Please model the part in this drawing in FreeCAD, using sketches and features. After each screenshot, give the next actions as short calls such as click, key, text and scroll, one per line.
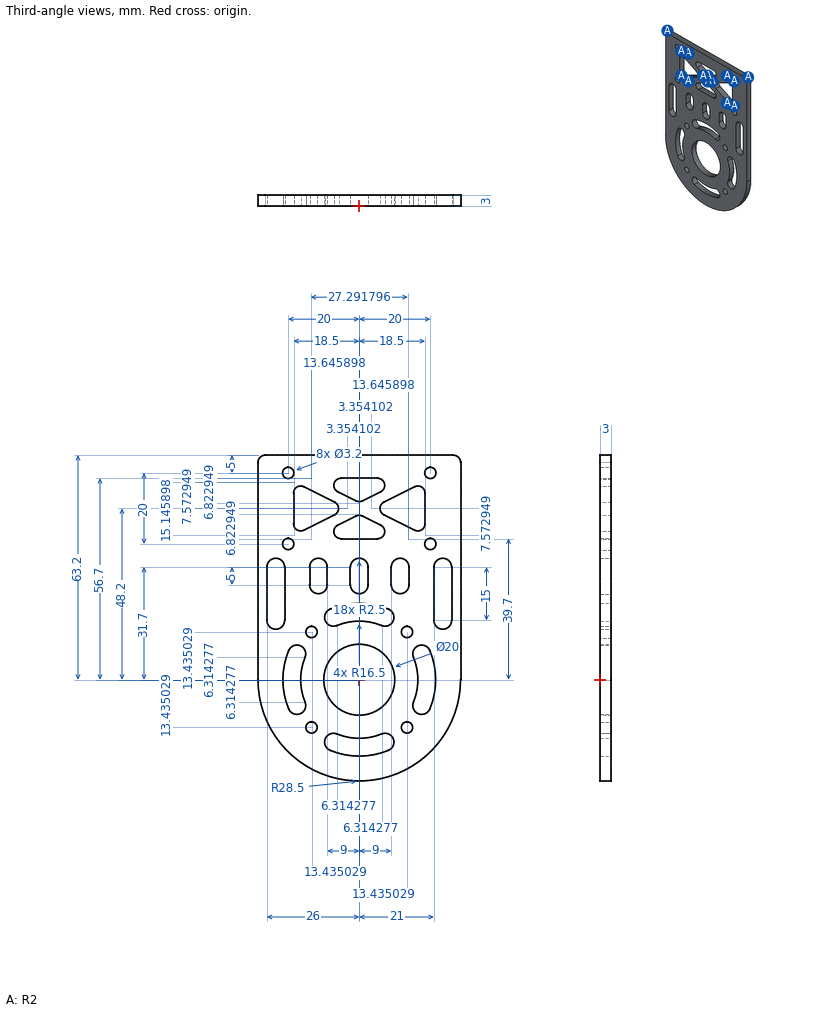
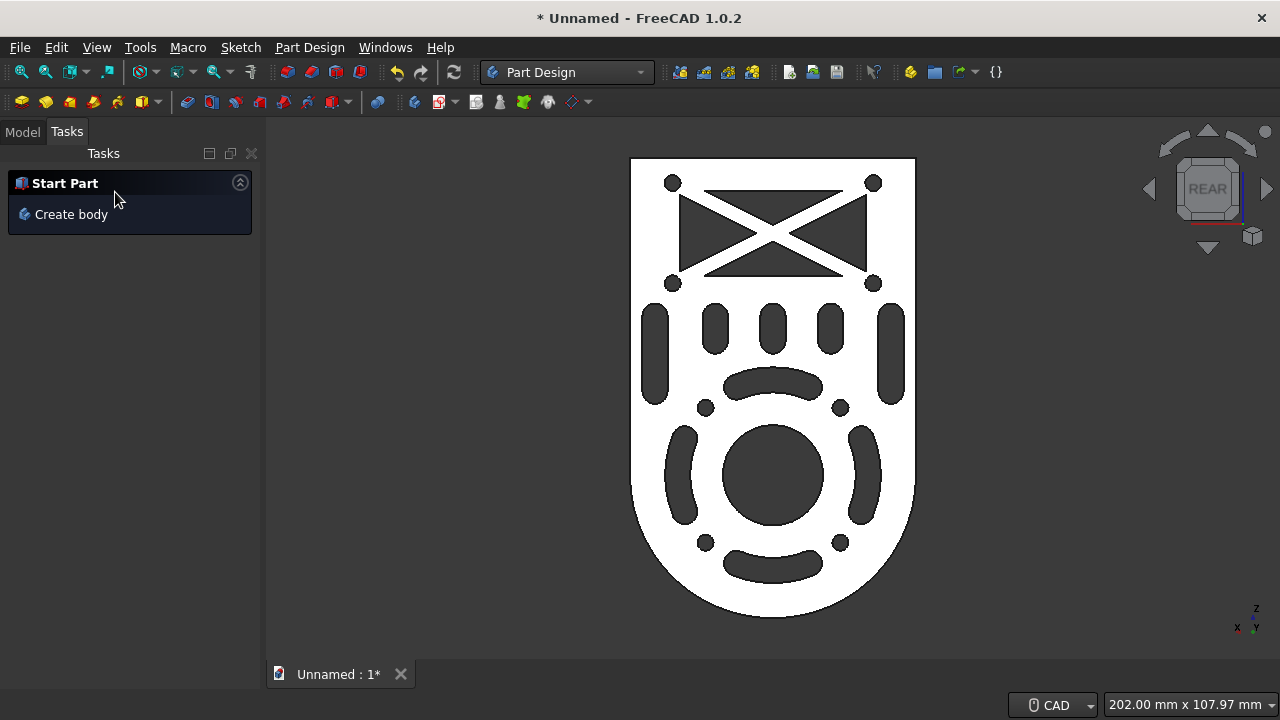
scroll(756, 232, up, 5)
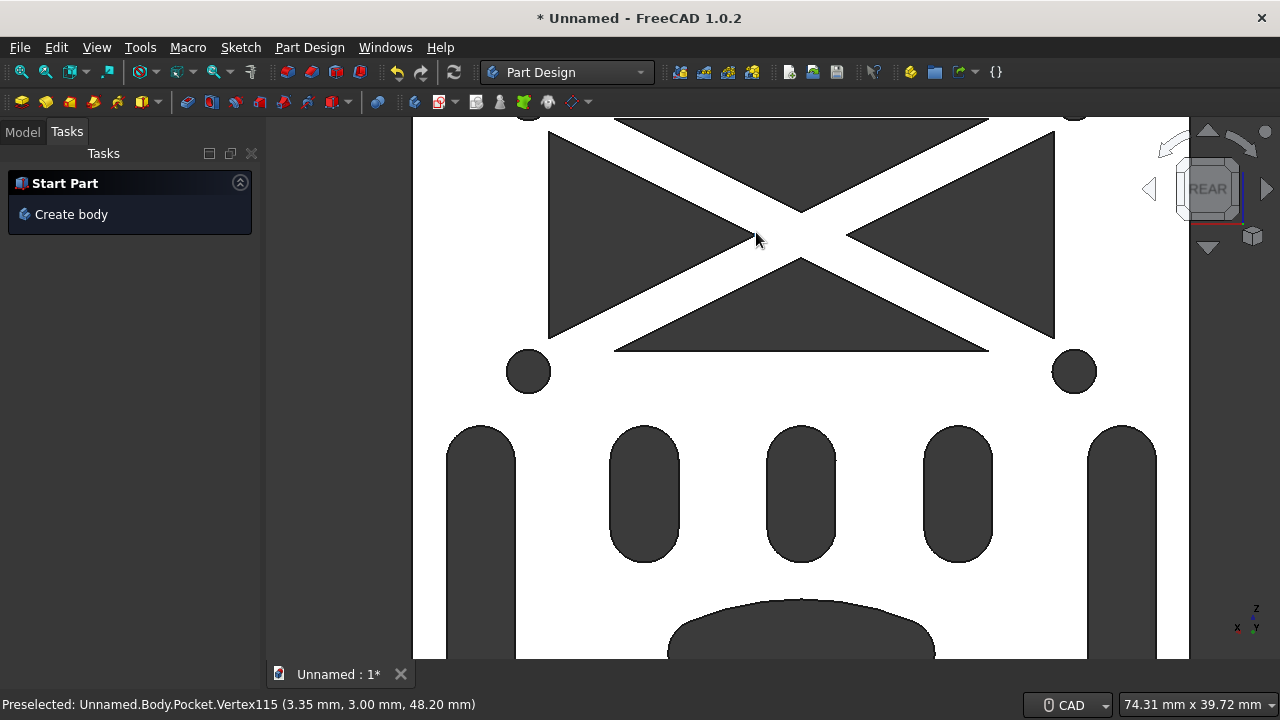
key(v)
key(f)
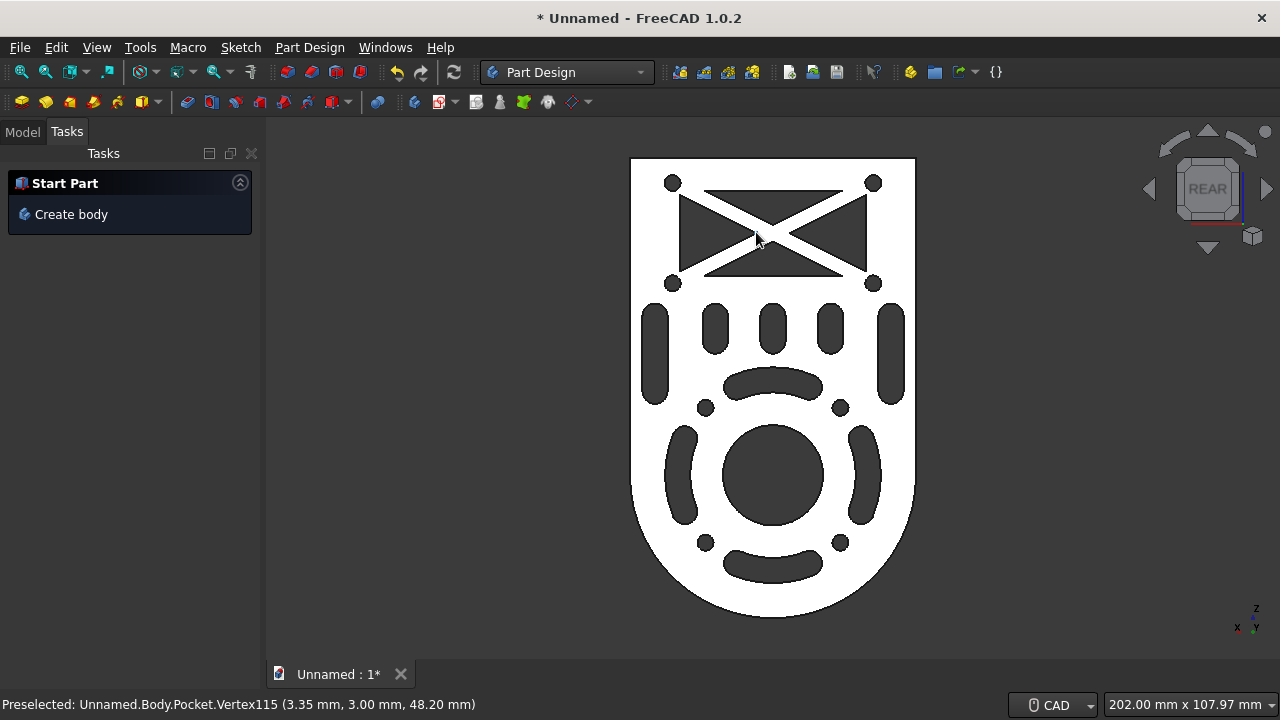
key(0)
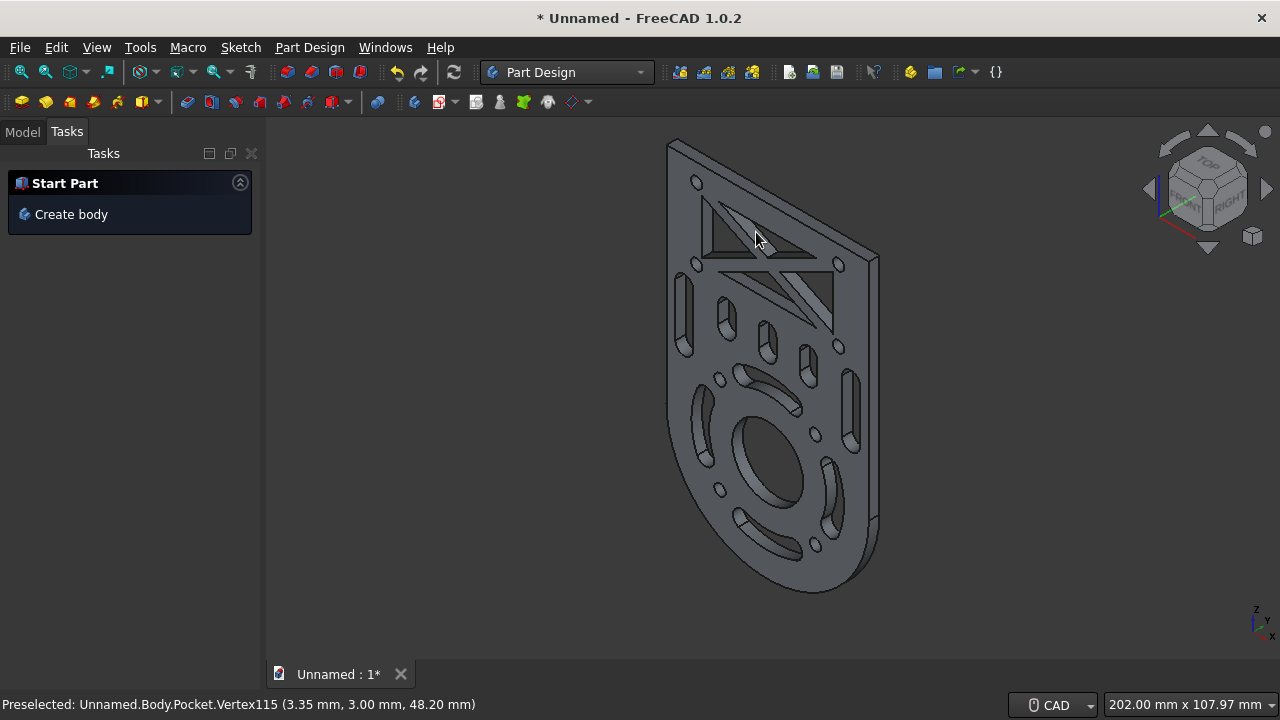
click(875, 257)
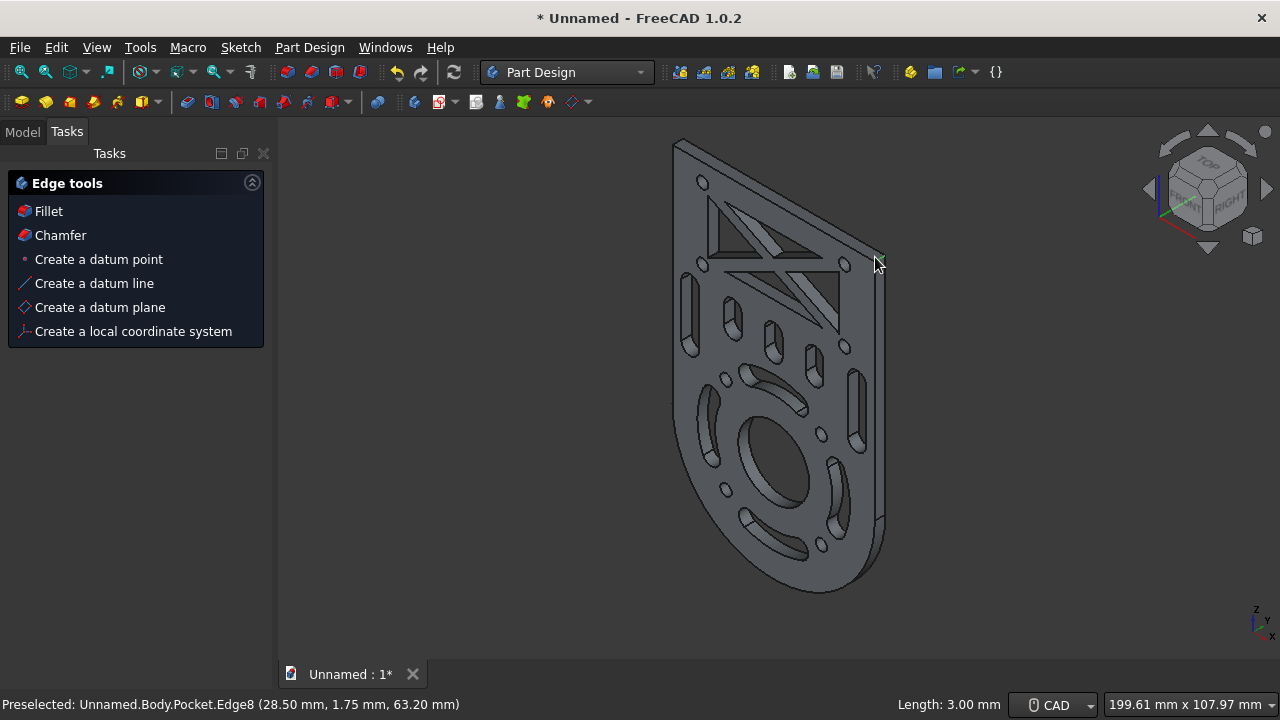
scroll(791, 268, up, 5)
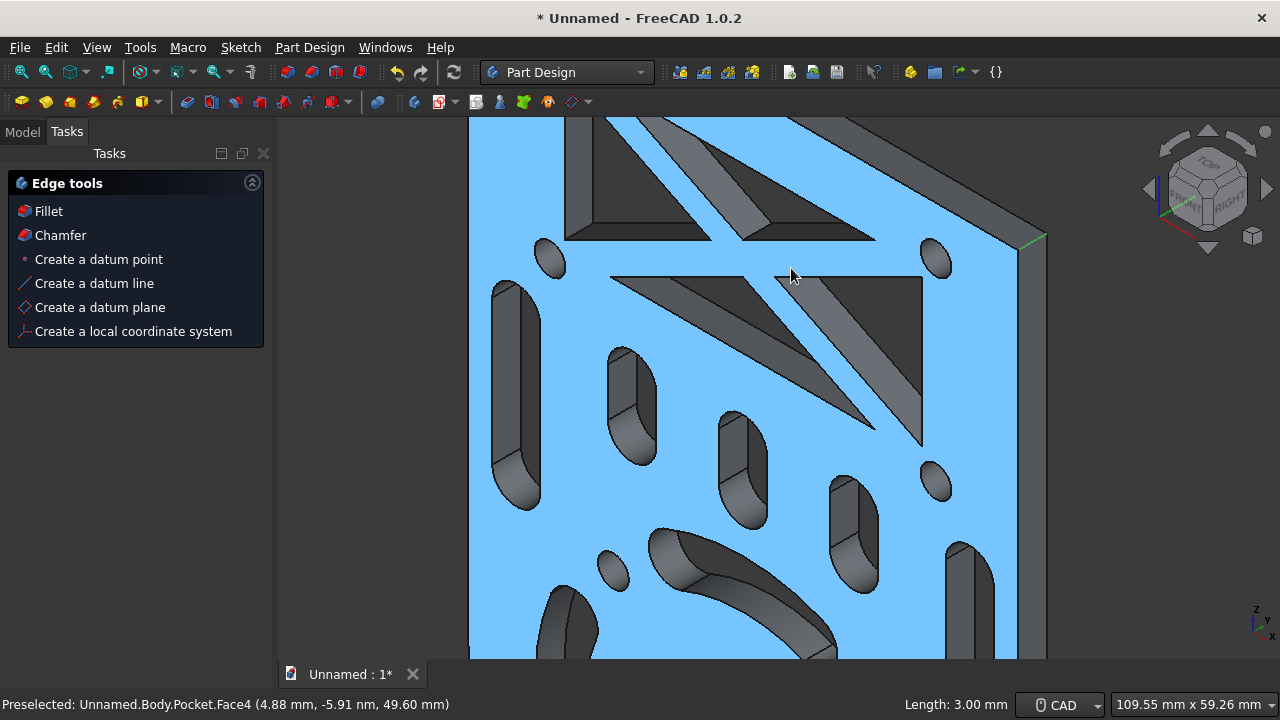
click(22, 72)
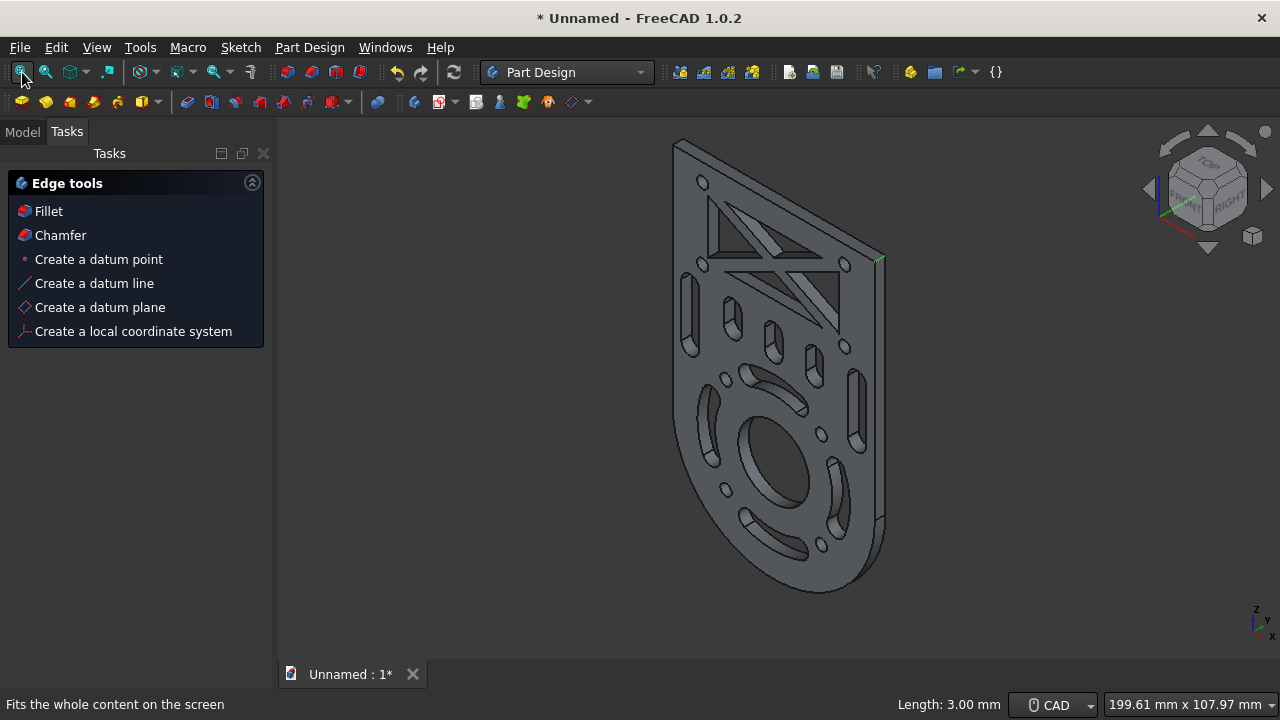
key(2)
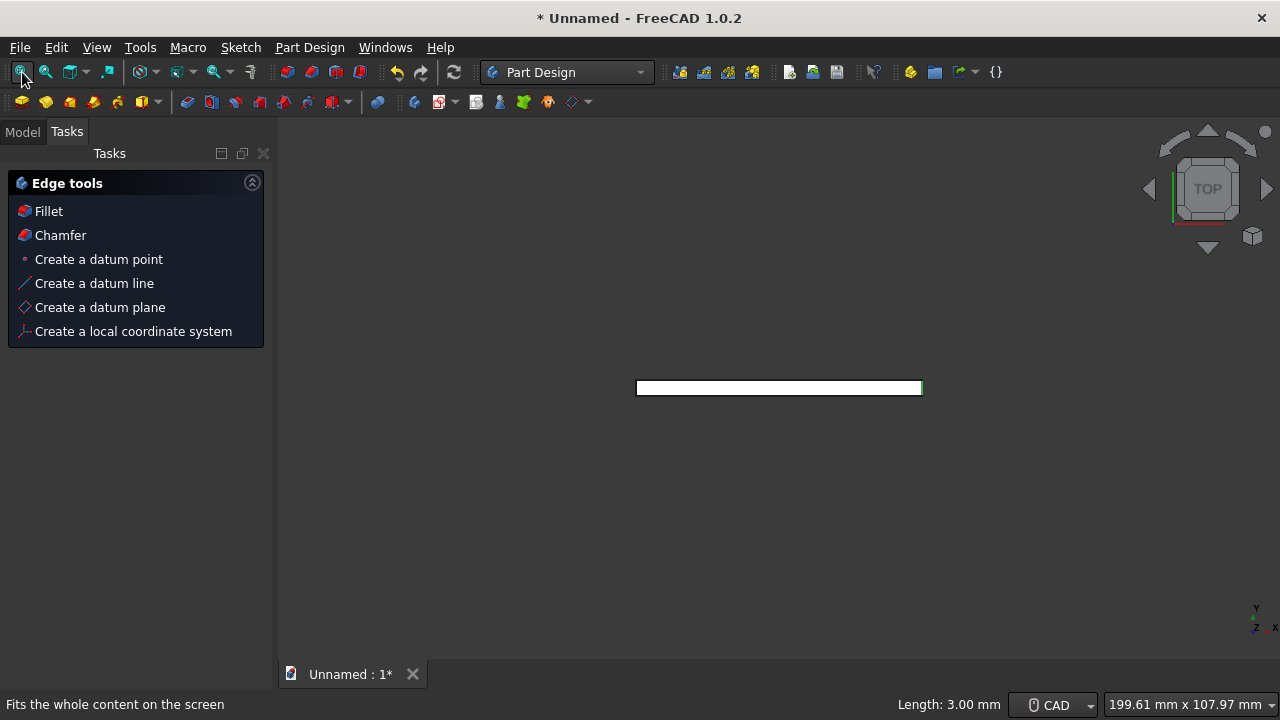
key(v)
key(f)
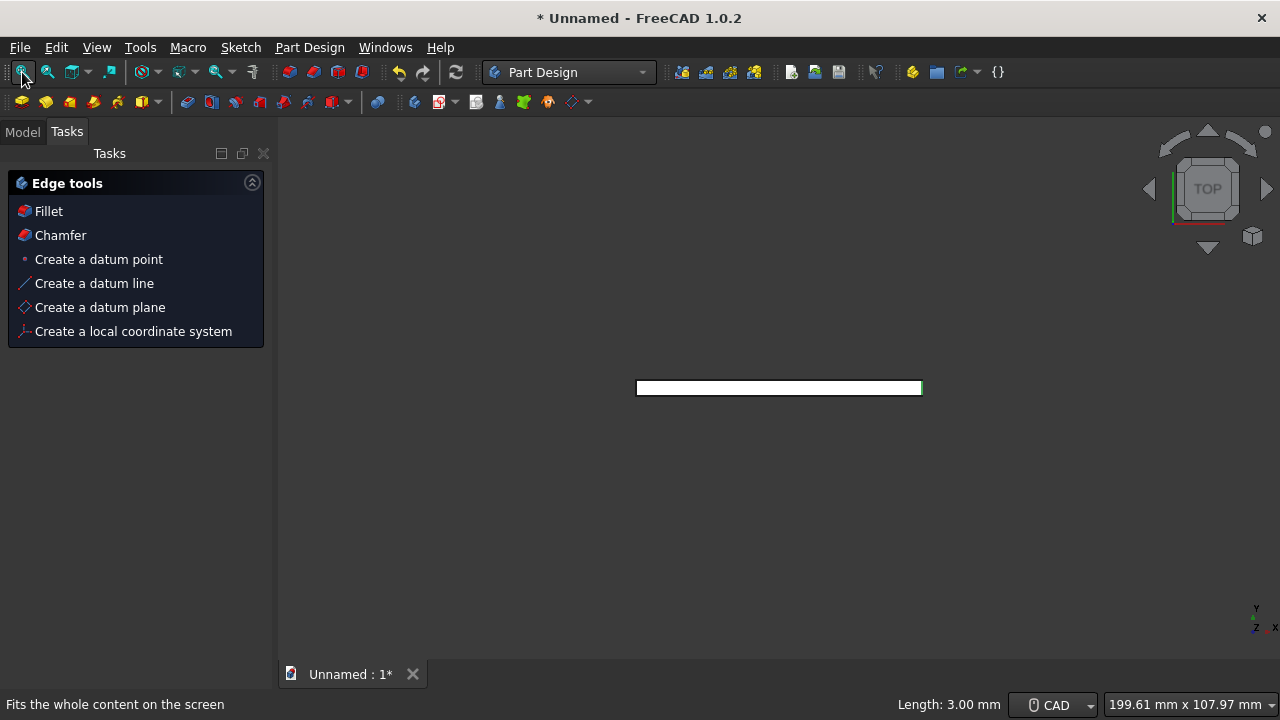
click(636, 387, ctrl)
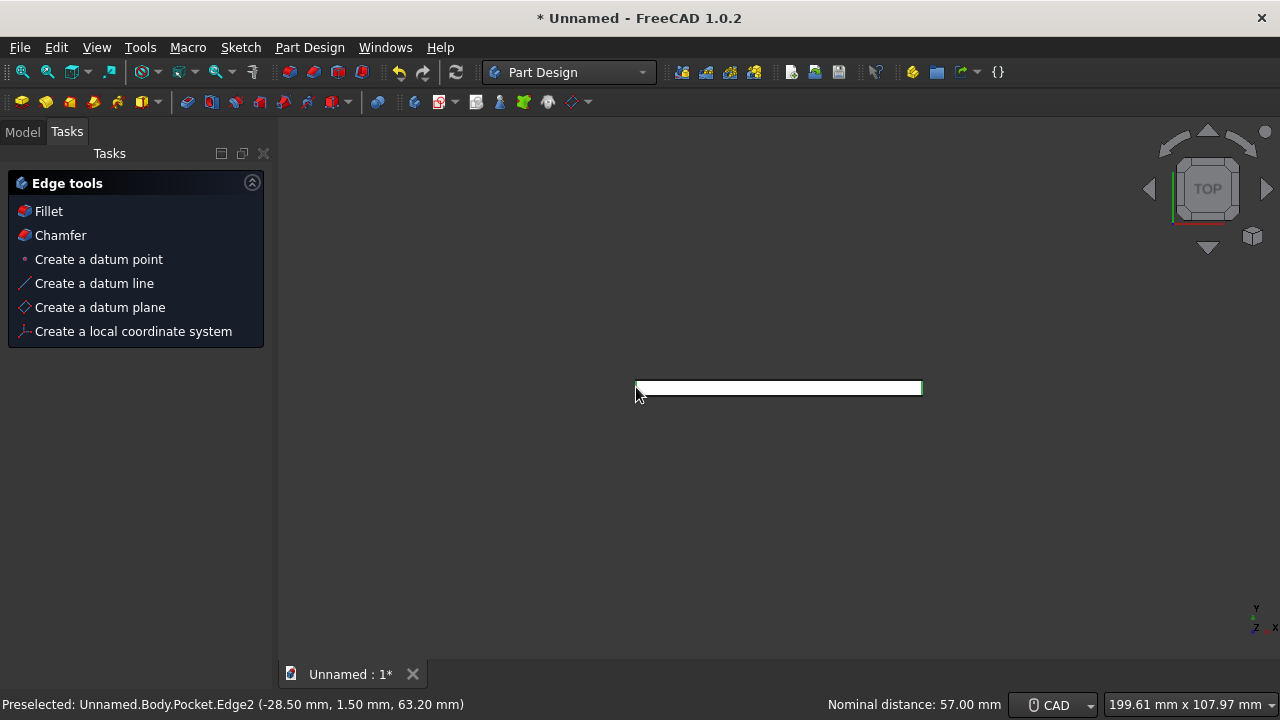
scroll(796, 387, up, 5)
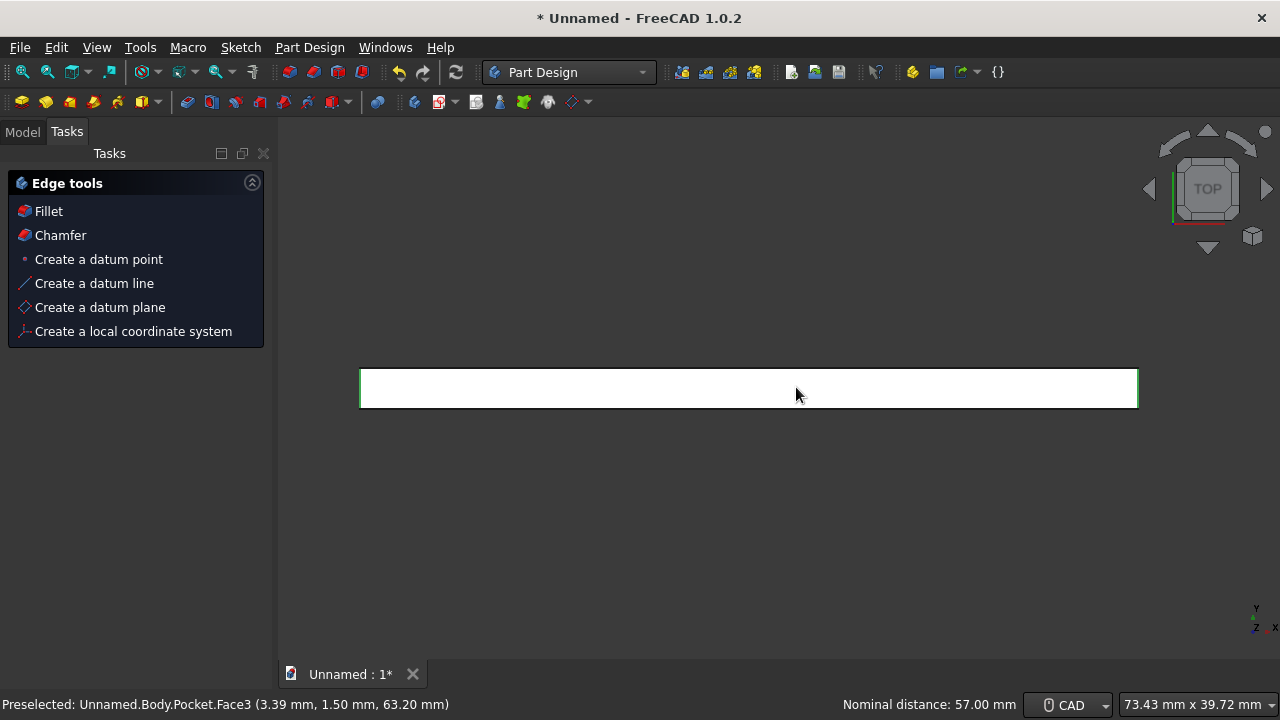
key(v)
key(f)